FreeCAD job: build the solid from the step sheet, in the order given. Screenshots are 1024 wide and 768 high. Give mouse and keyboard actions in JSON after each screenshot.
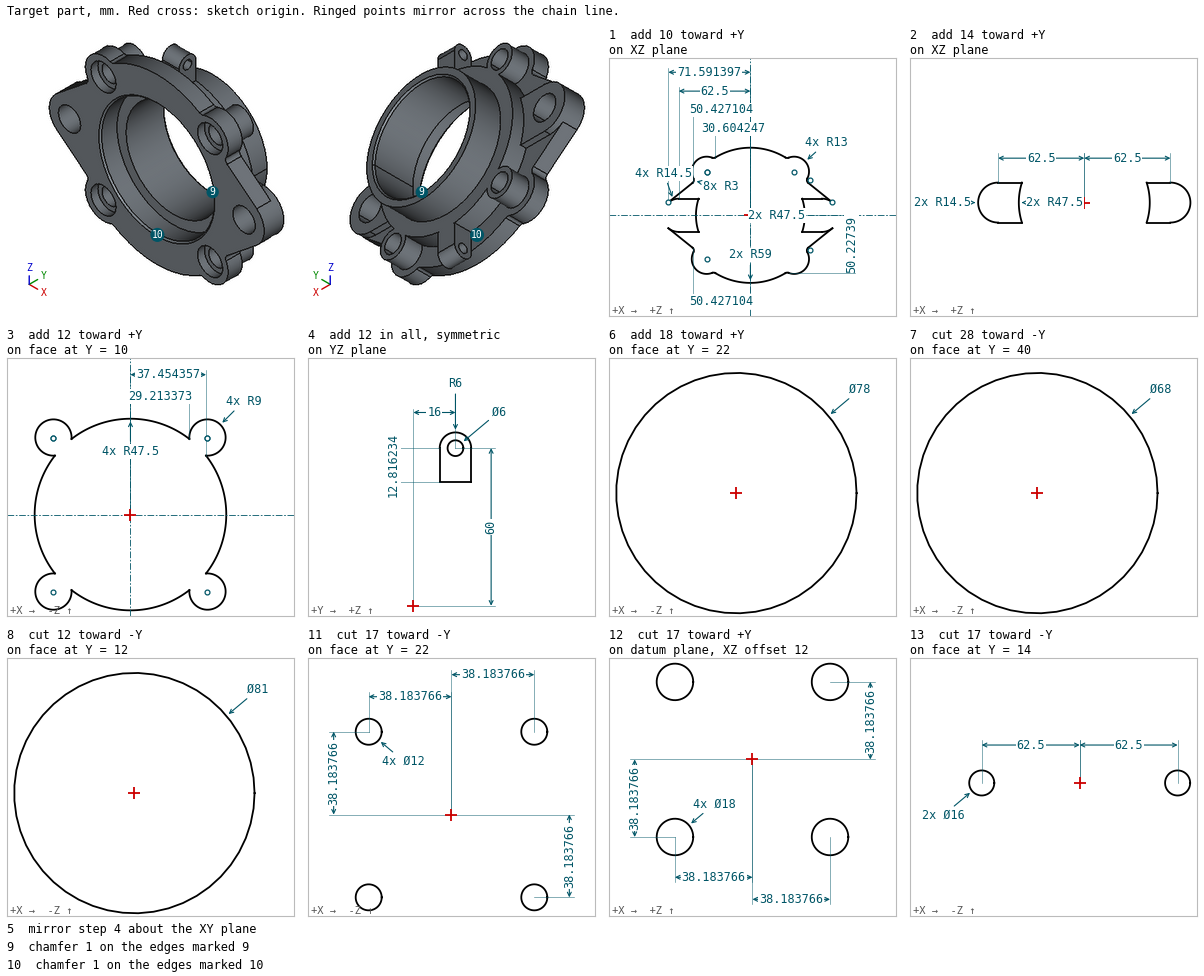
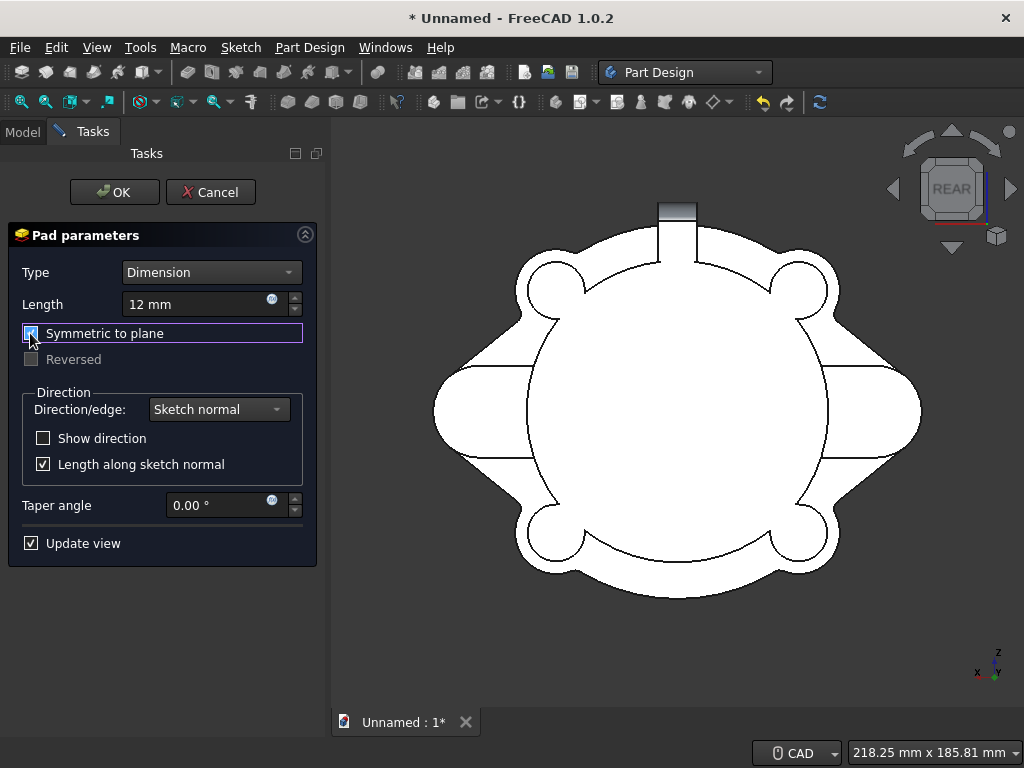
{"action": "left_click", "coordinate": [115, 192]}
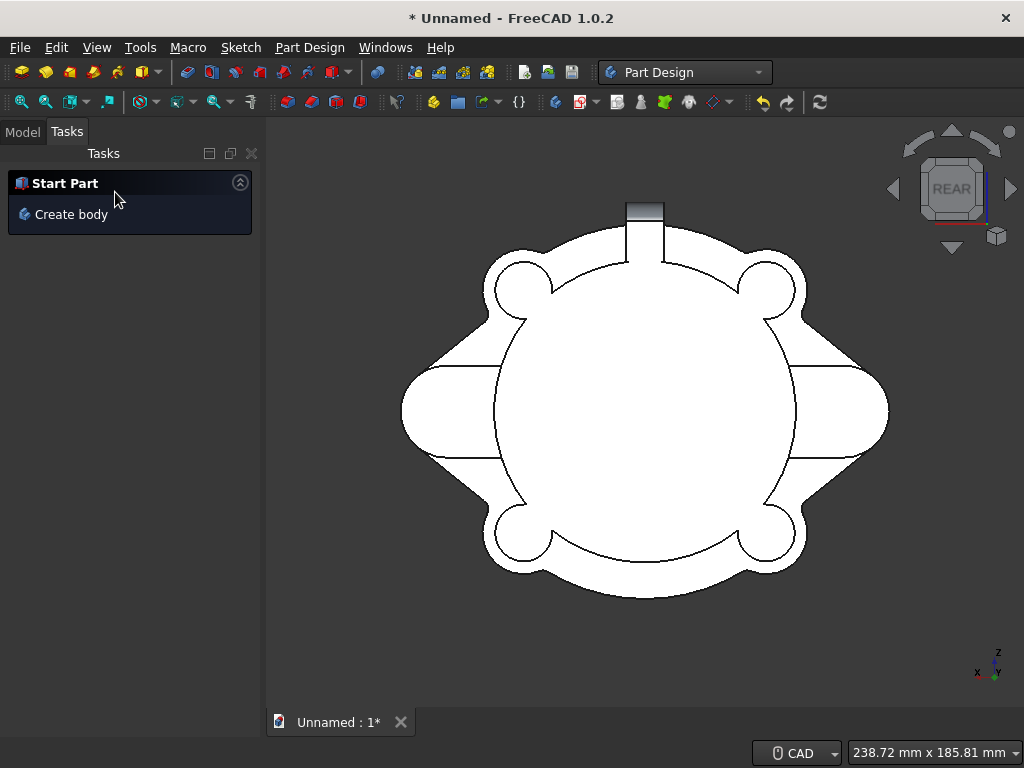
{"action": "left_click", "coordinate": [23, 131]}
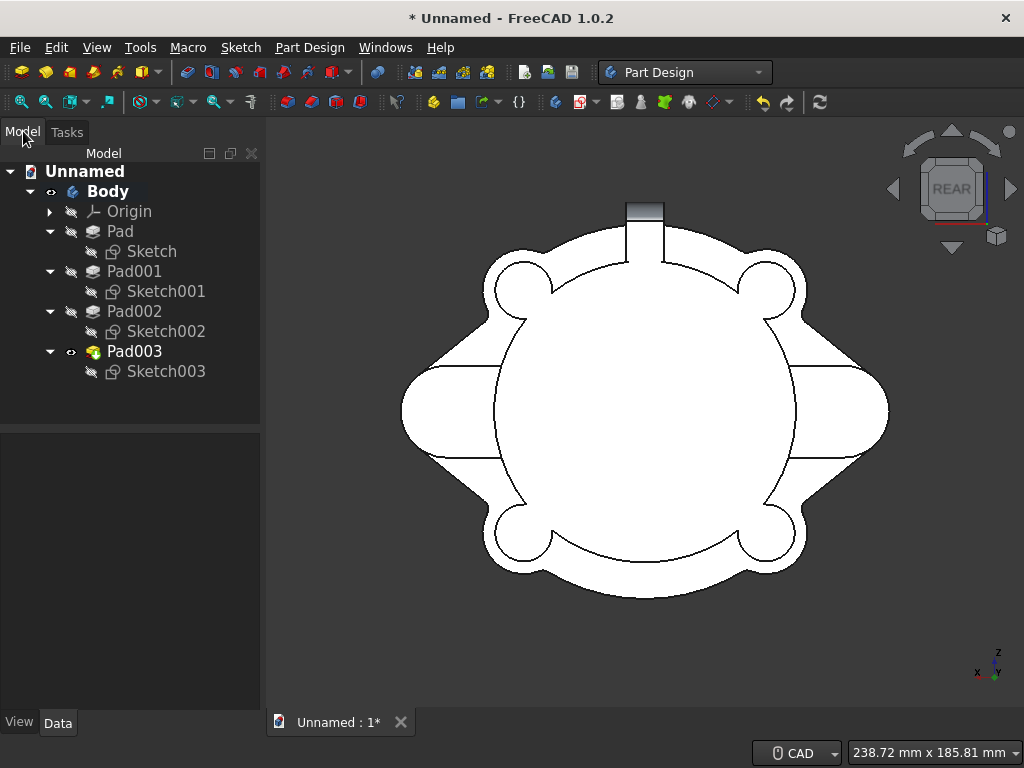
{"action": "left_click", "coordinate": [116, 352]}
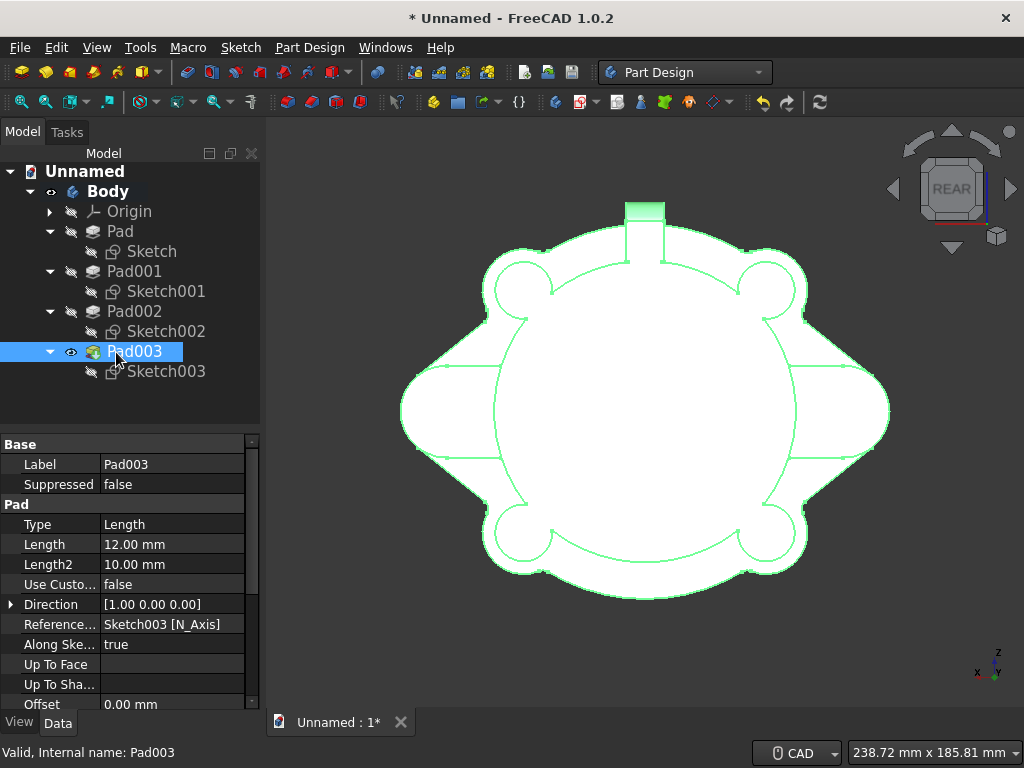
{"action": "left_click", "coordinate": [416, 72]}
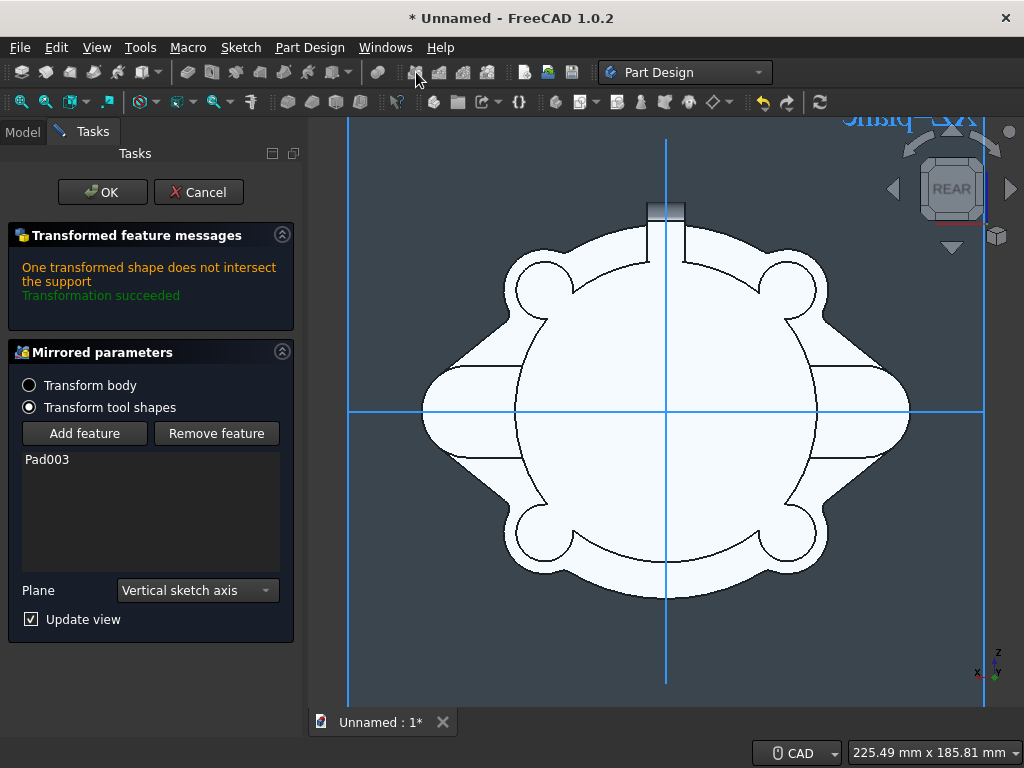
{"action": "left_click", "coordinate": [198, 590]}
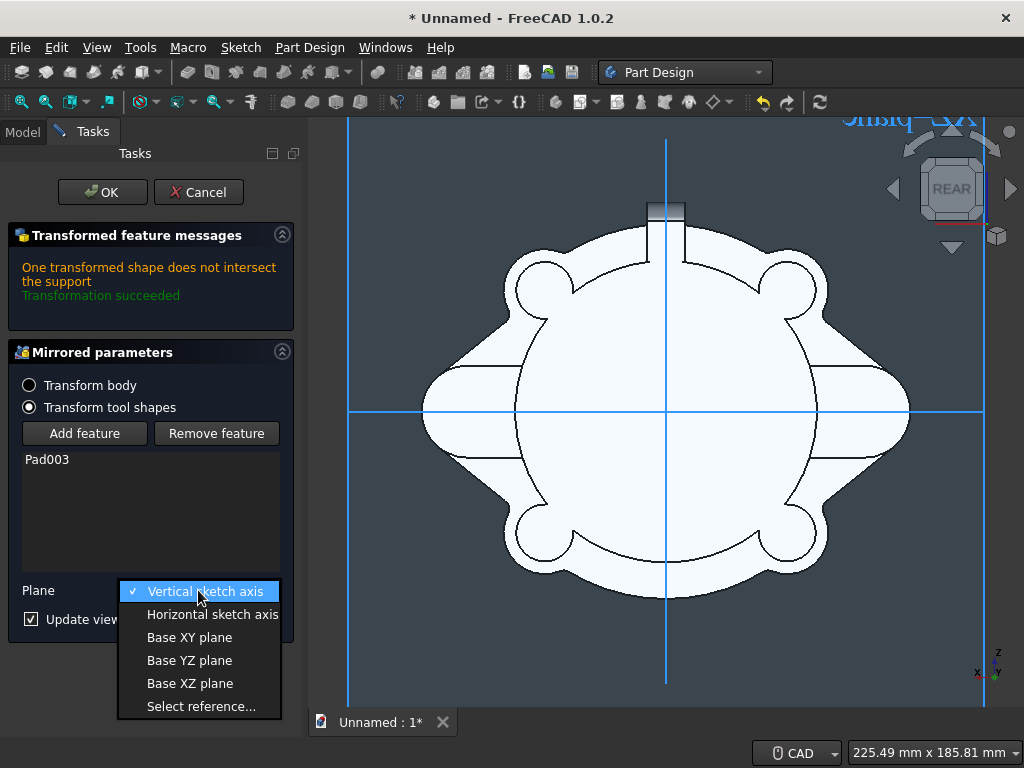
{"action": "left_click", "coordinate": [198, 638]}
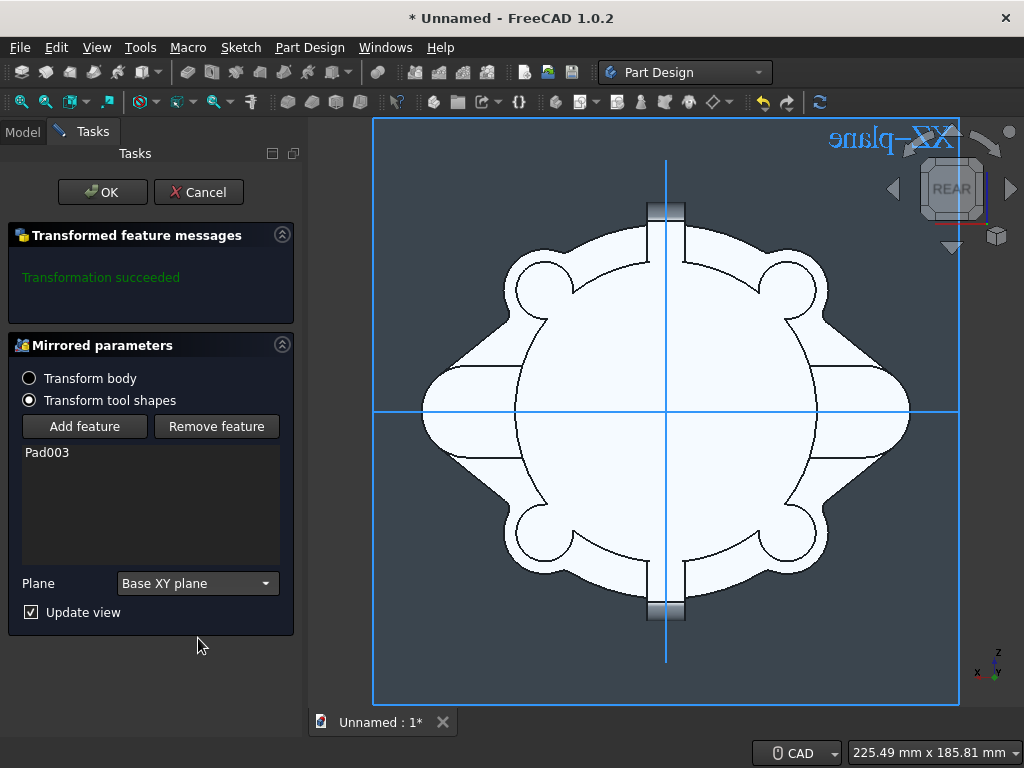
{"action": "left_click", "coordinate": [103, 192]}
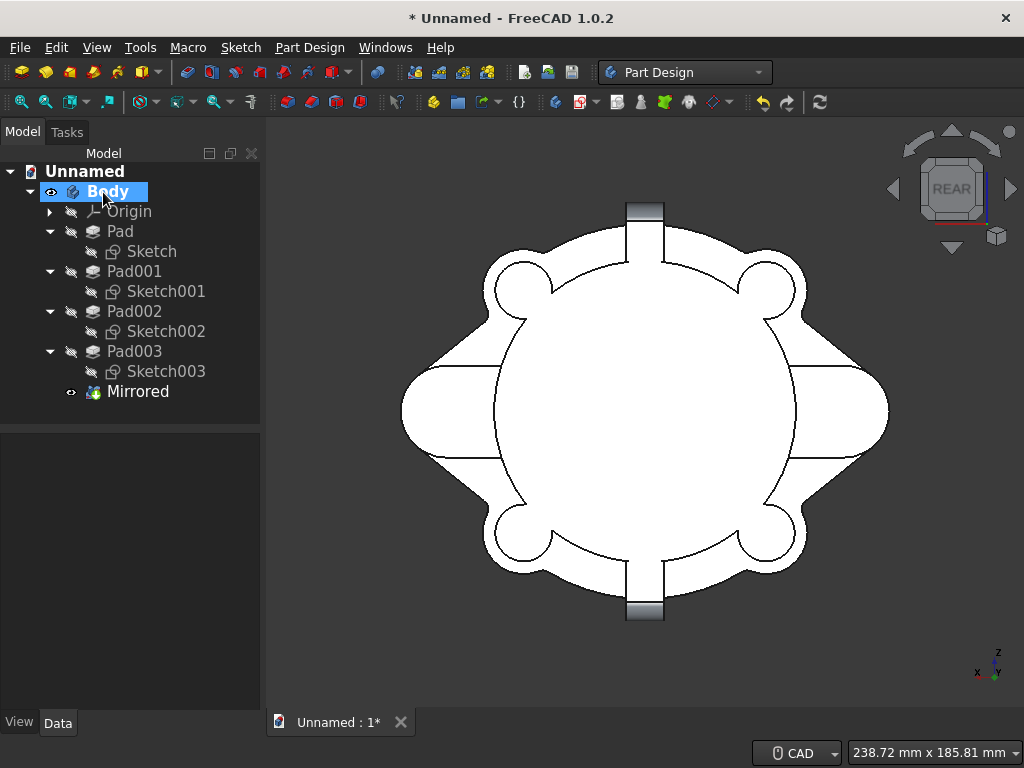
{"action": "left_click", "coordinate": [645, 411]}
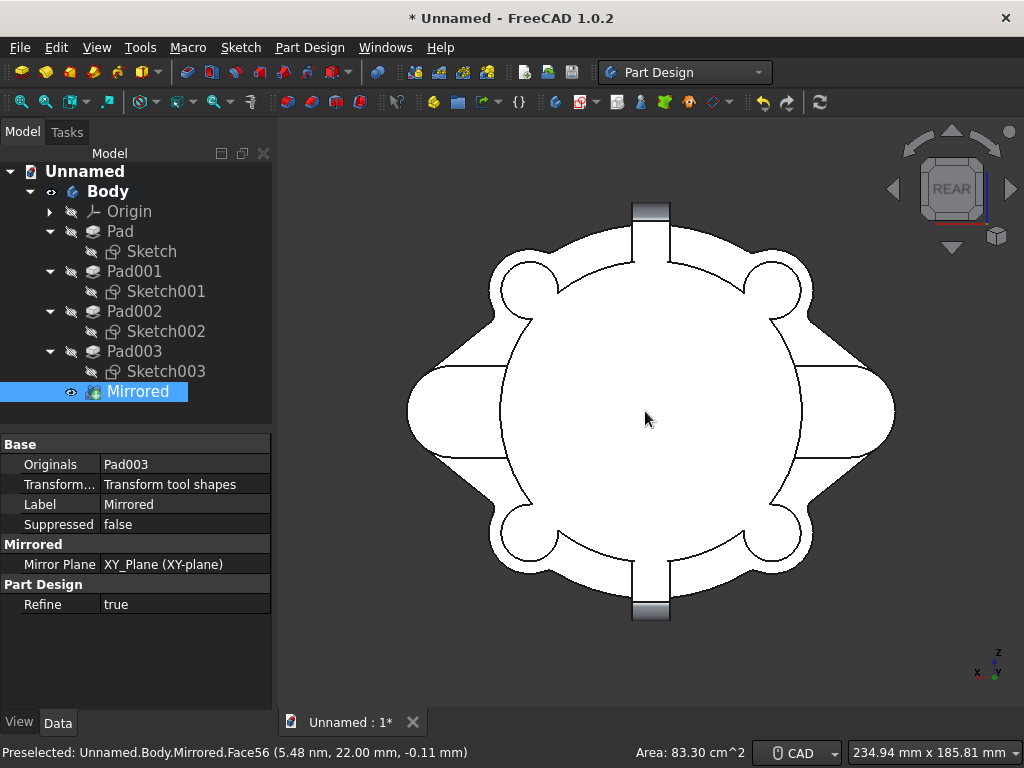
{"action": "left_click", "coordinate": [580, 102]}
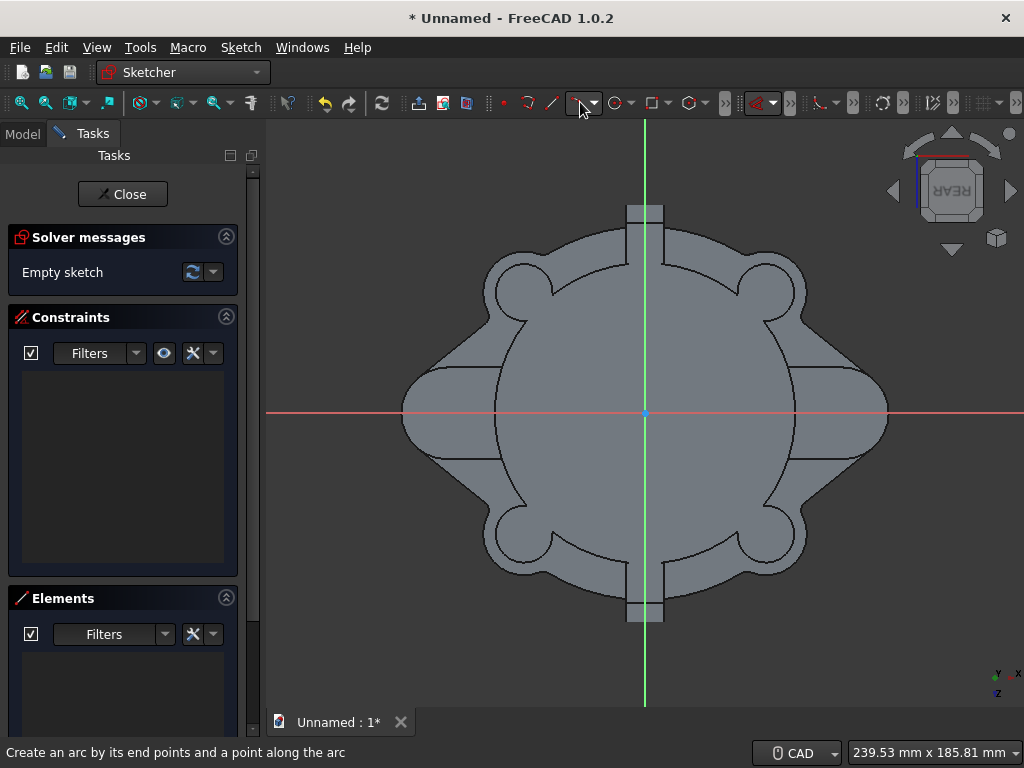
{"action": "scroll", "coordinate": [784, 414], "scroll_direction": "up", "scroll_amount": 2}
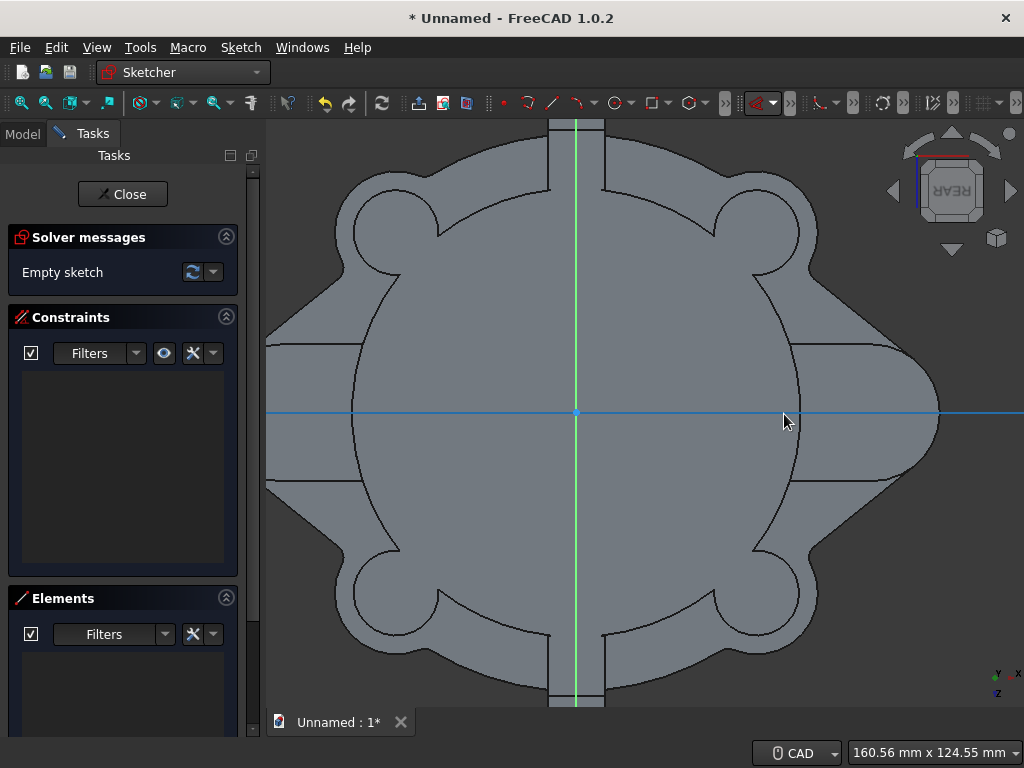
{"action": "key", "text": "g c"}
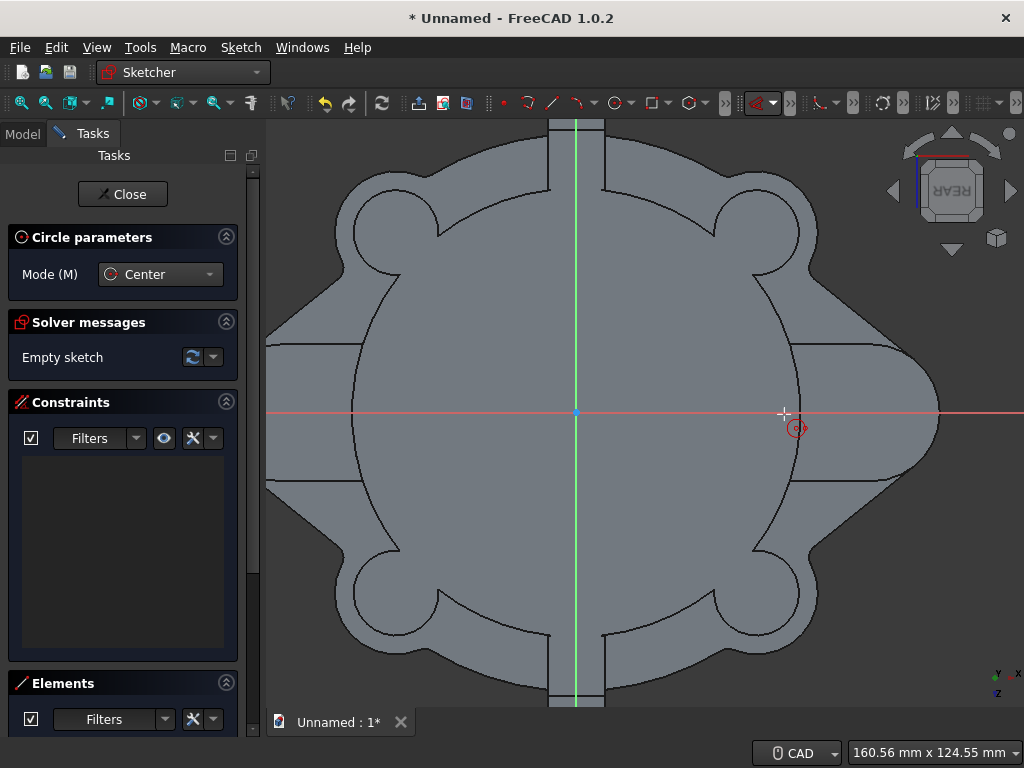
{"action": "left_click", "coordinate": [576, 413]}
{"action": "left_click", "coordinate": [706, 283]}
{"action": "key", "text": "Escape"}